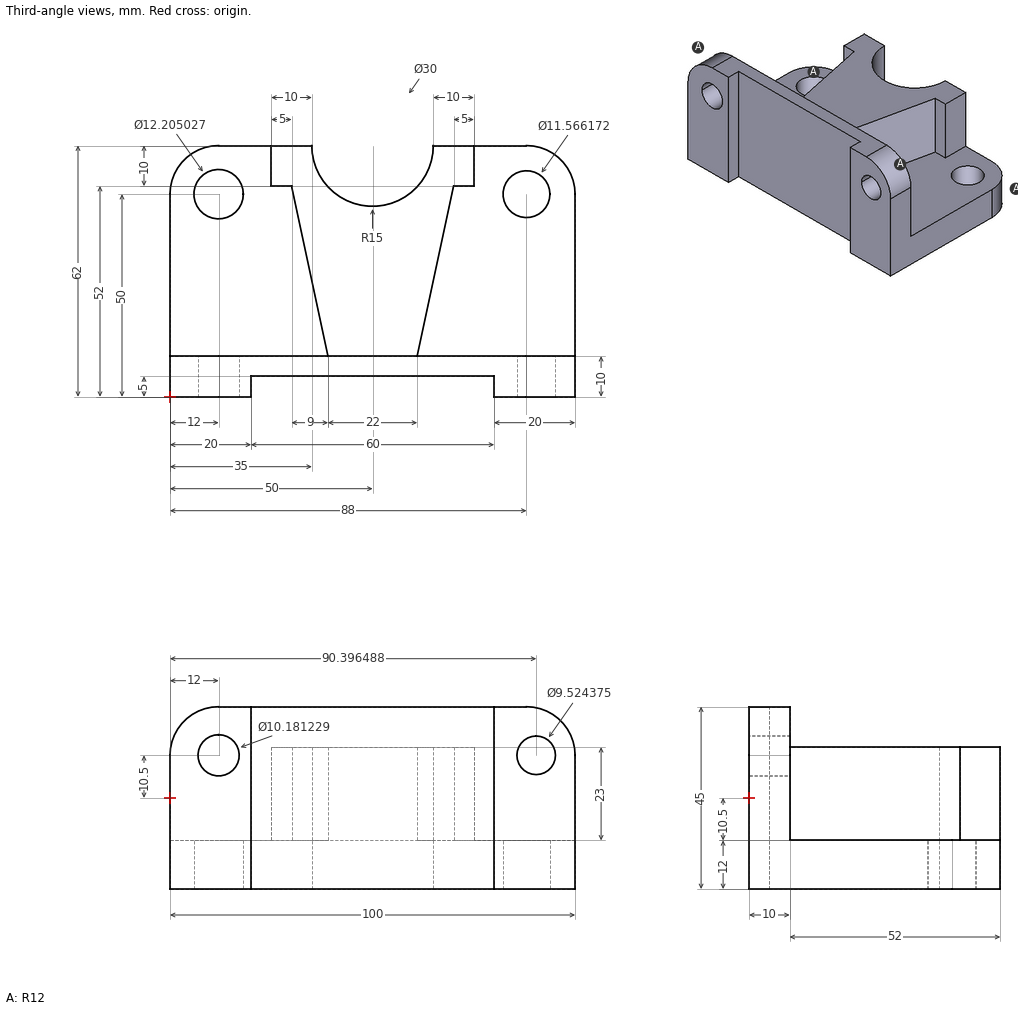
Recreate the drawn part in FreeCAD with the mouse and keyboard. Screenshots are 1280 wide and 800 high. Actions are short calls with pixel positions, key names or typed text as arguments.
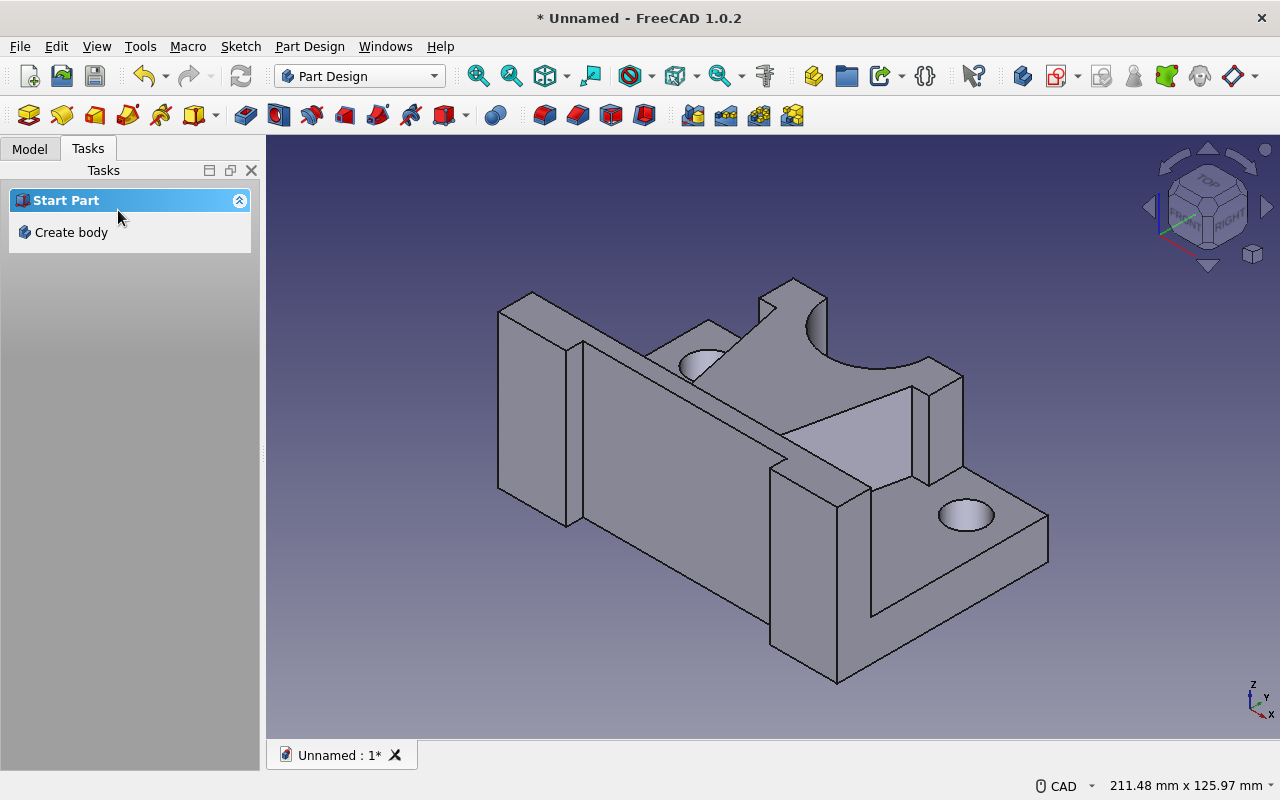
click(854, 497)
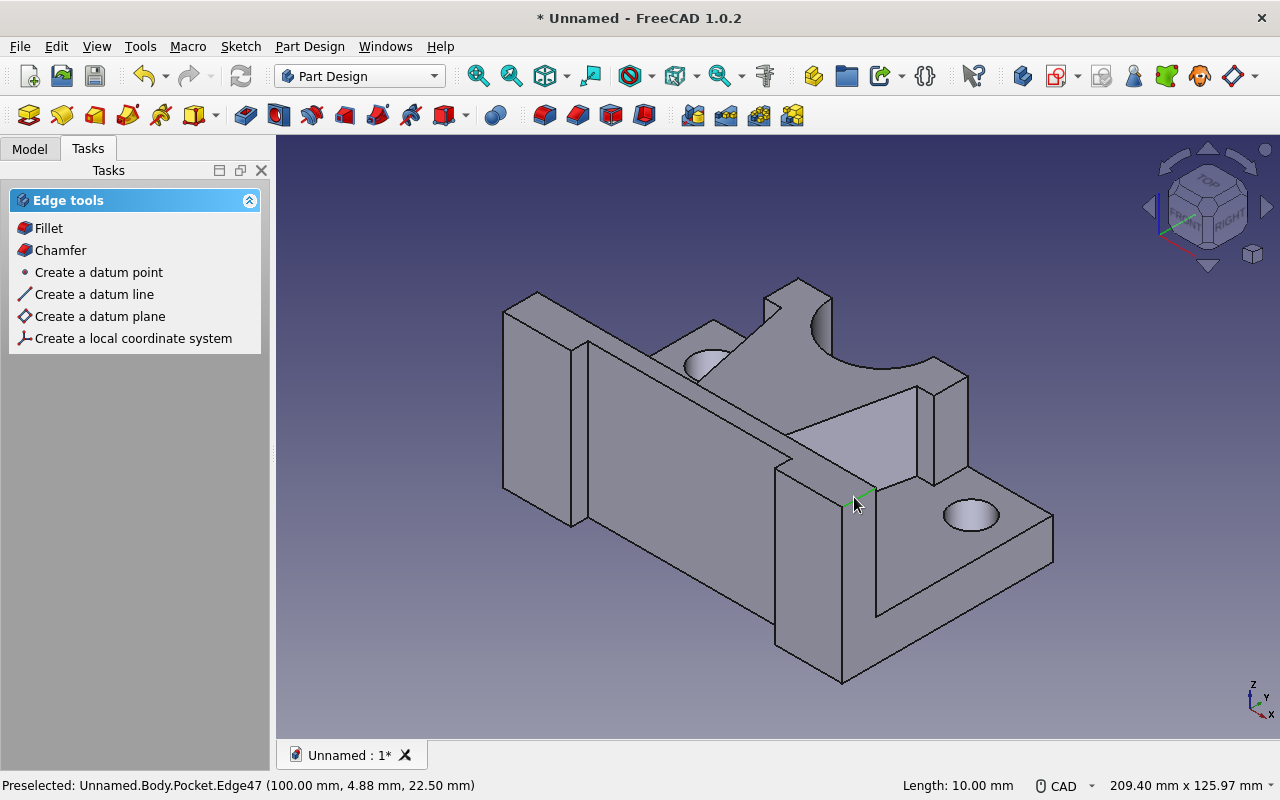
key(2)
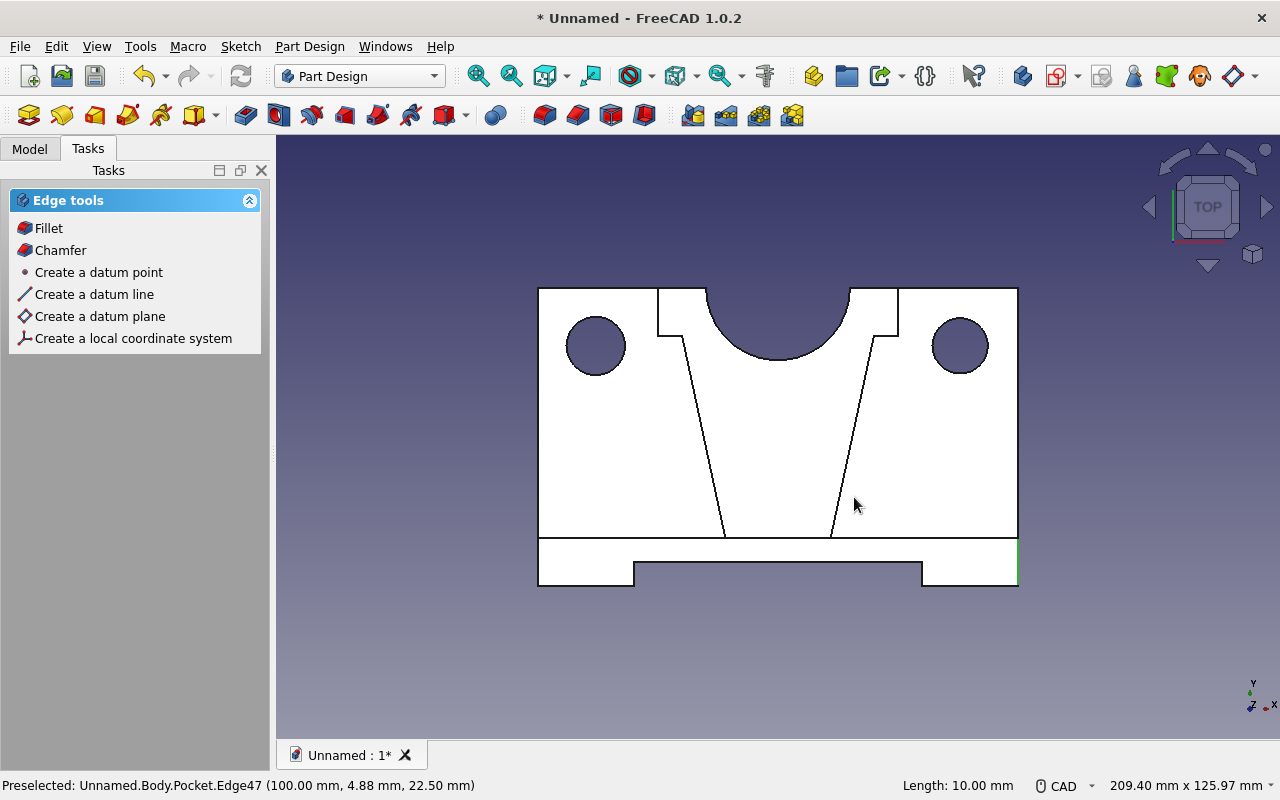
click(538, 561, ctrl)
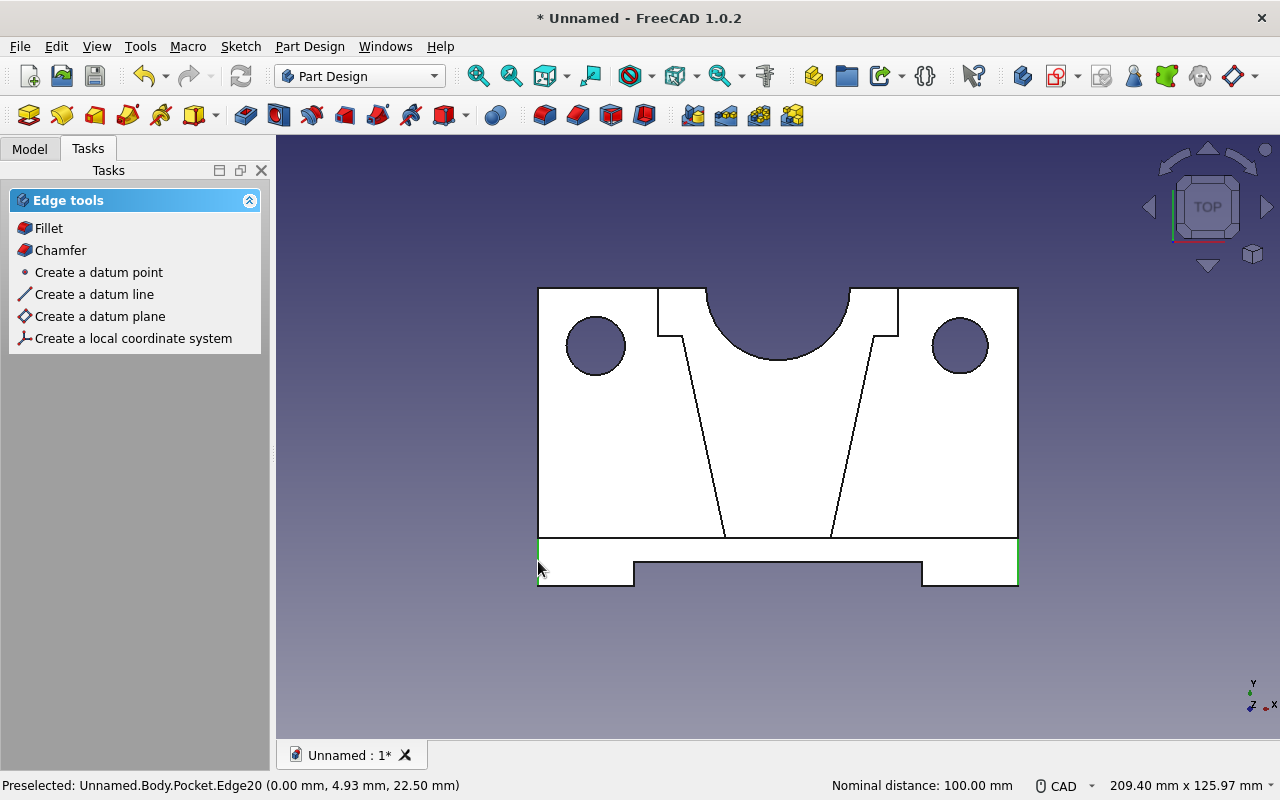
key(0)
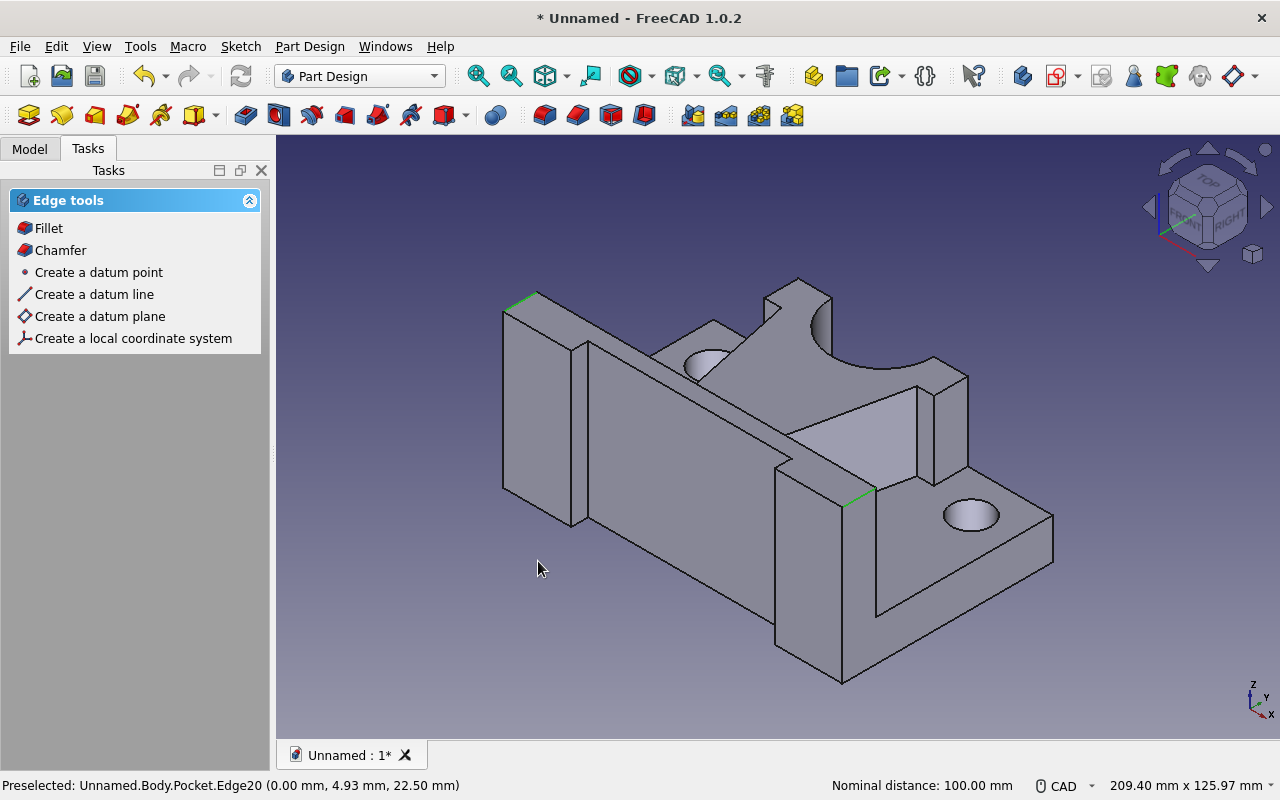
key(1)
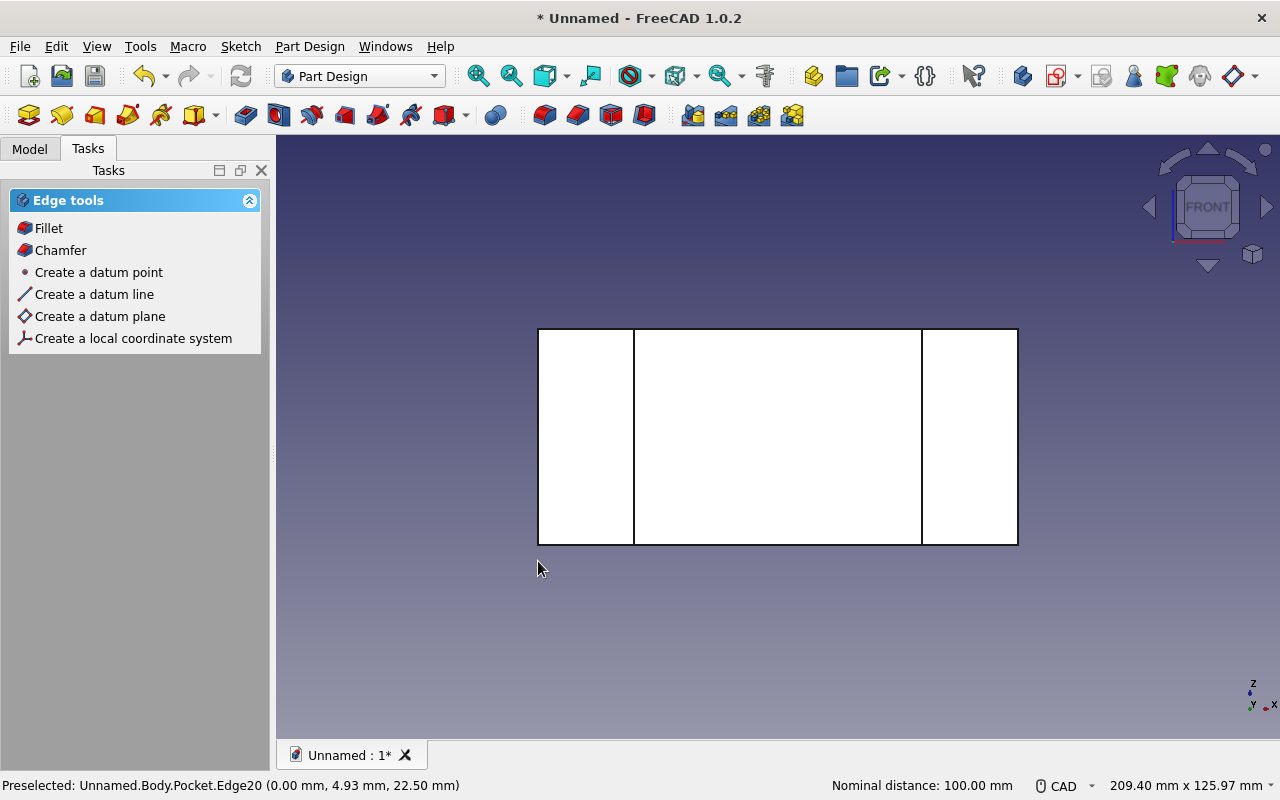
key(3)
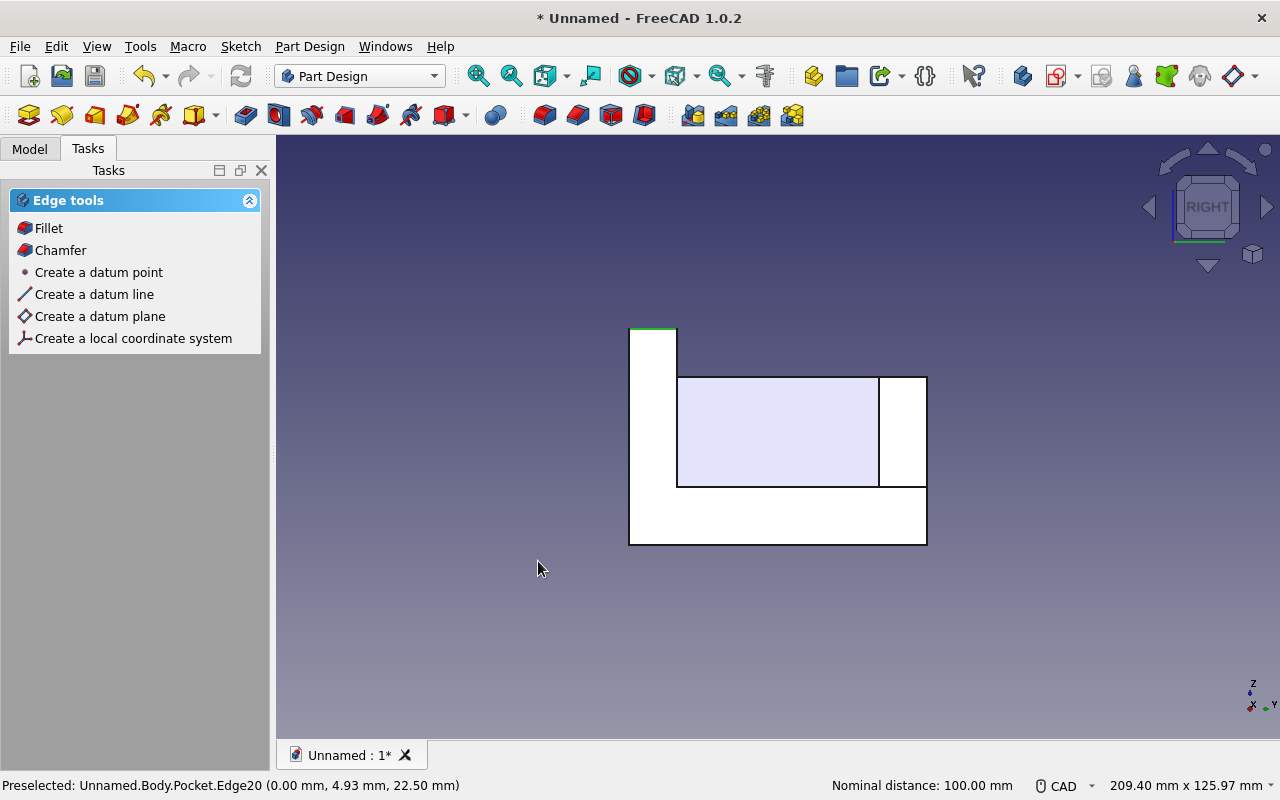
click(479, 76)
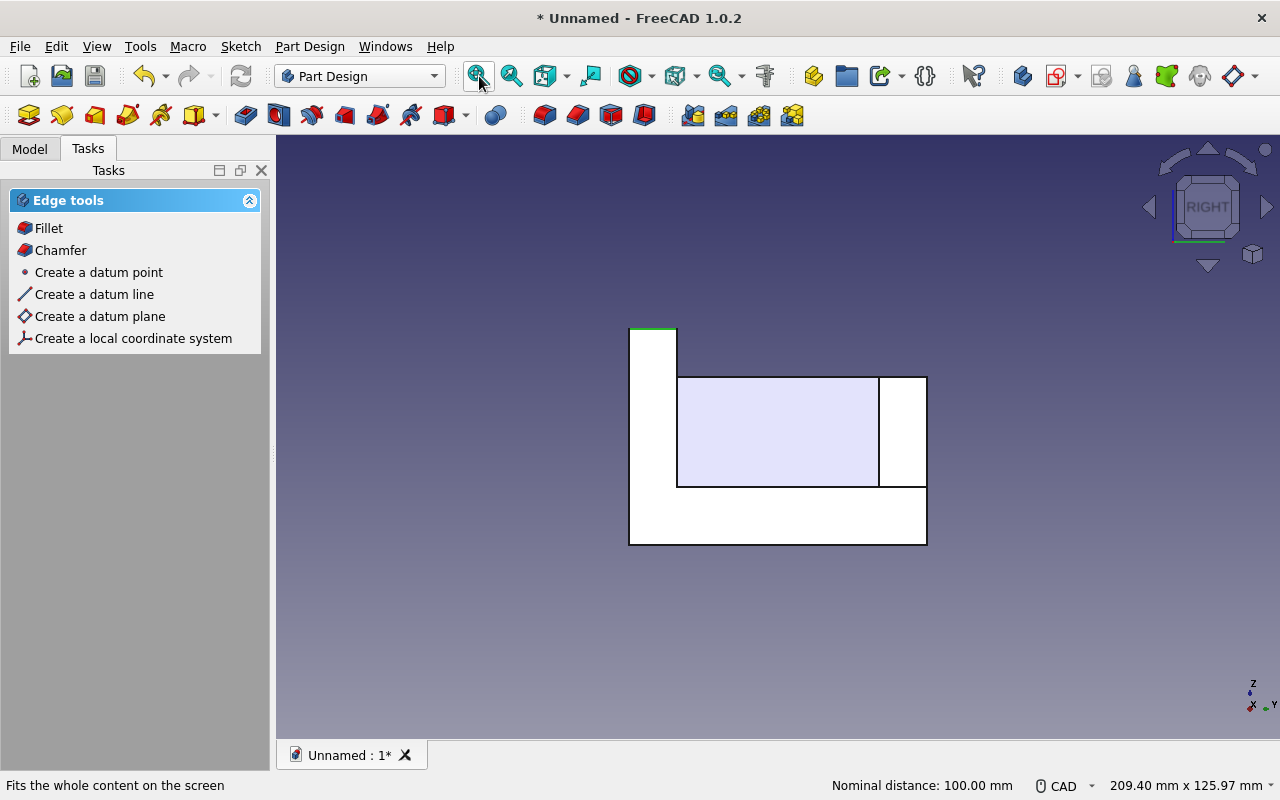
click(927, 515, ctrl)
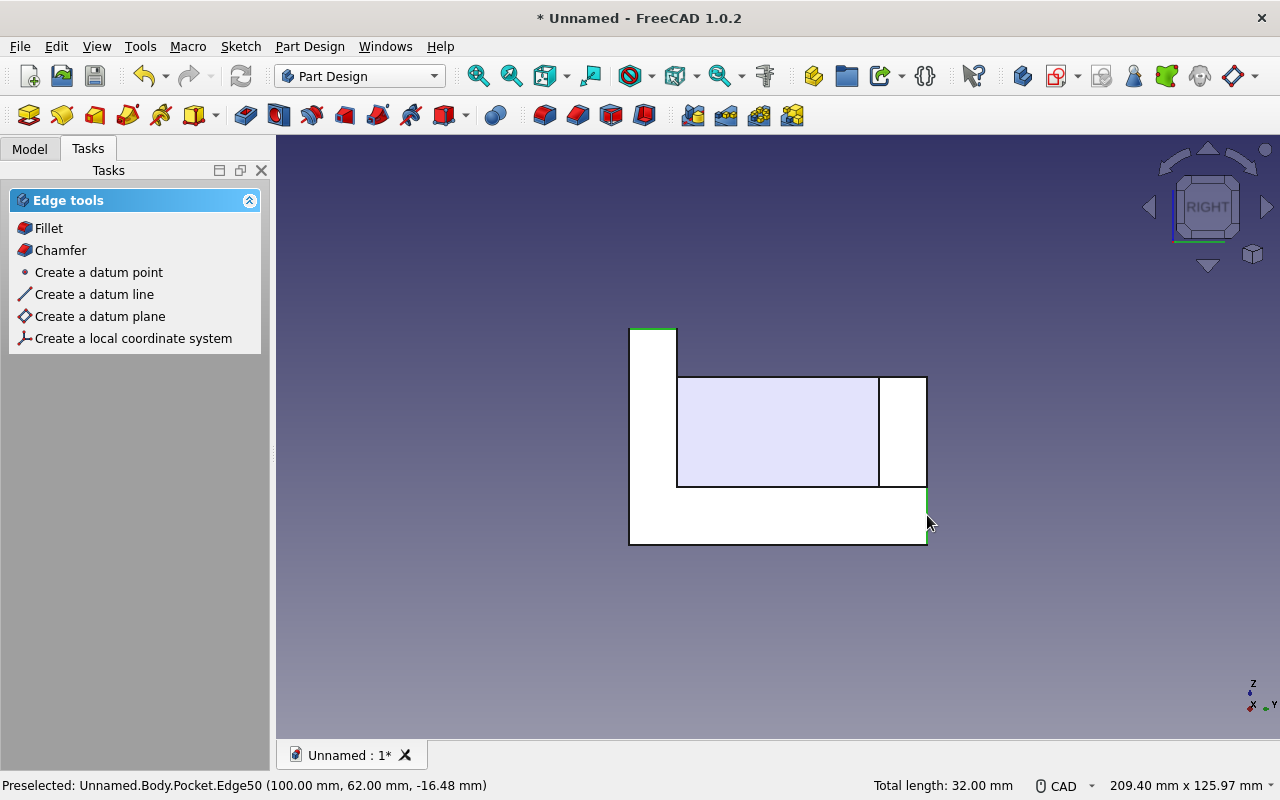
key(5)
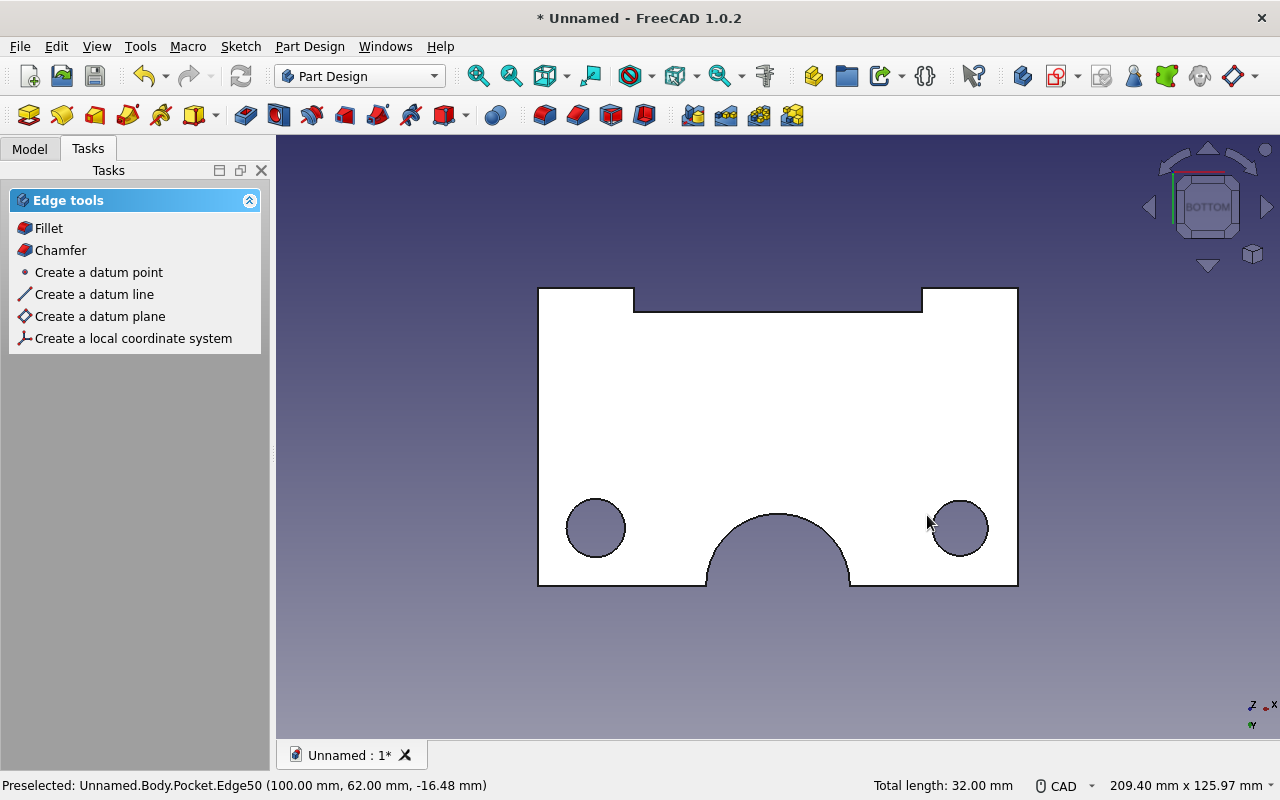
key(4)